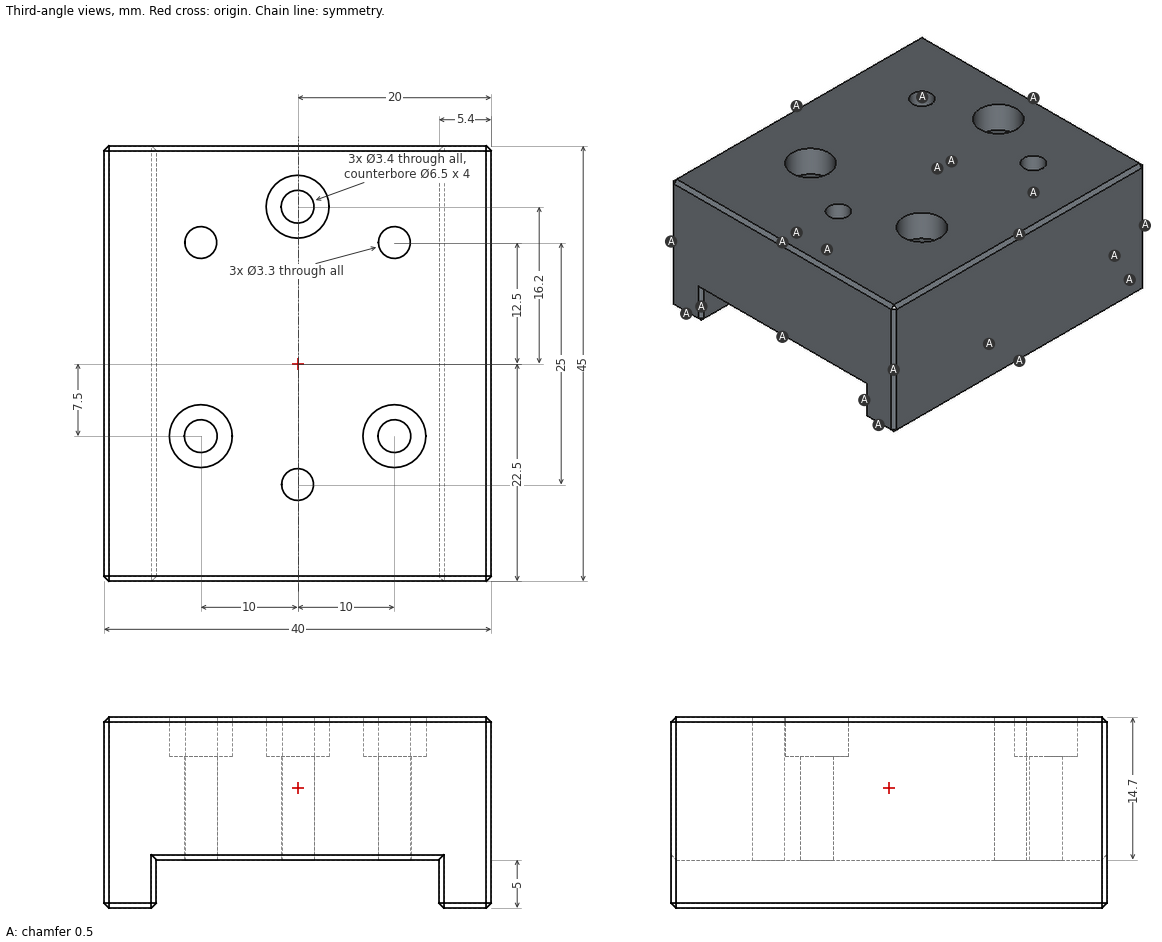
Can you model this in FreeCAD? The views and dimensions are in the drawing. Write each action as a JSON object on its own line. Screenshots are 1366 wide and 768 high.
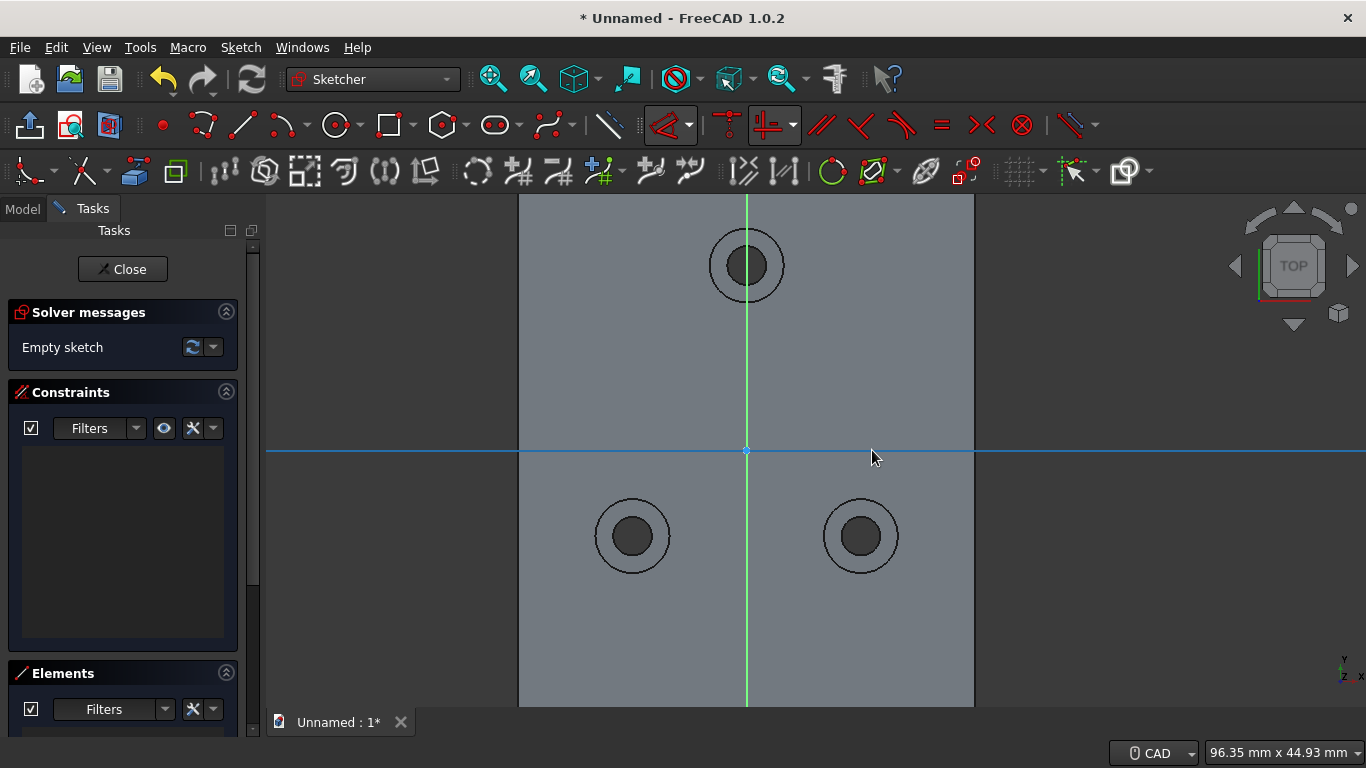
{"action": "left_click", "coordinate": [336, 126]}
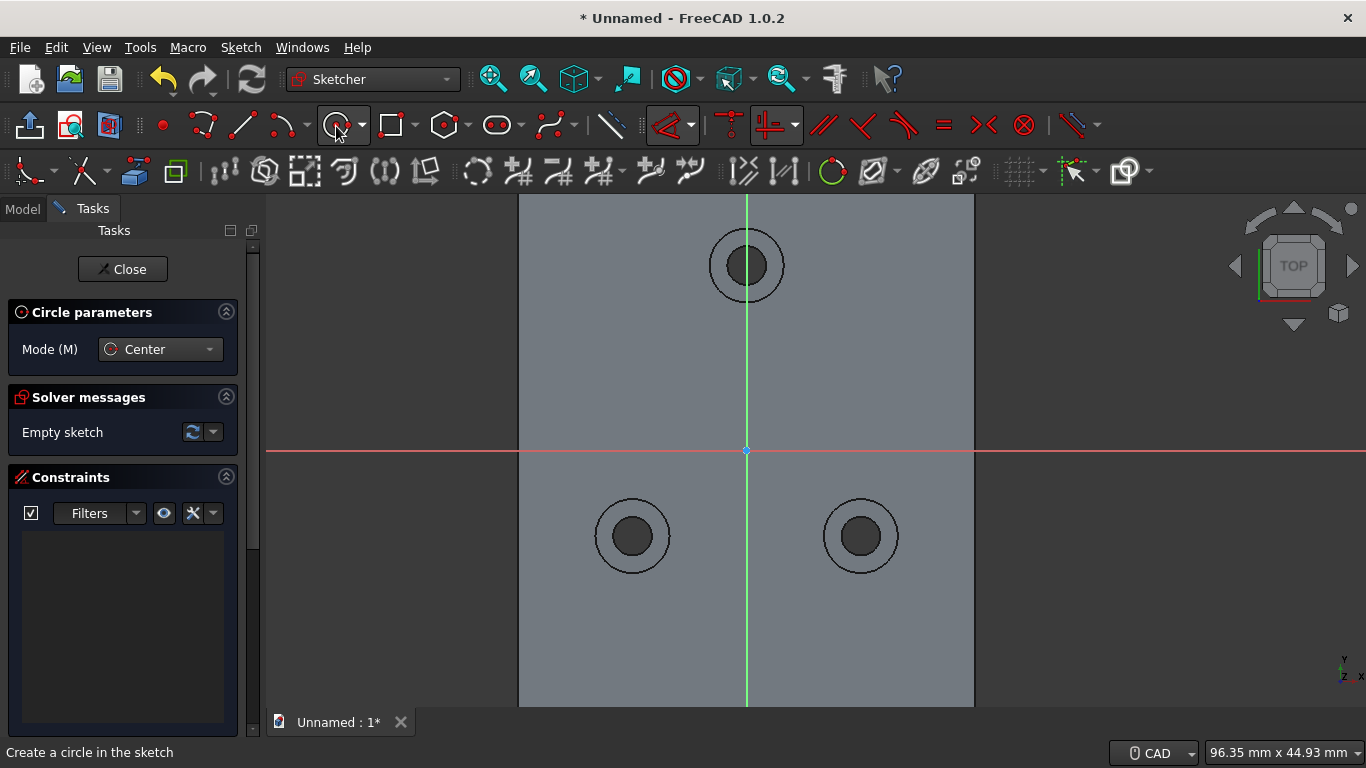
{"action": "left_click", "coordinate": [861, 308]}
{"action": "left_click", "coordinate": [874, 294]}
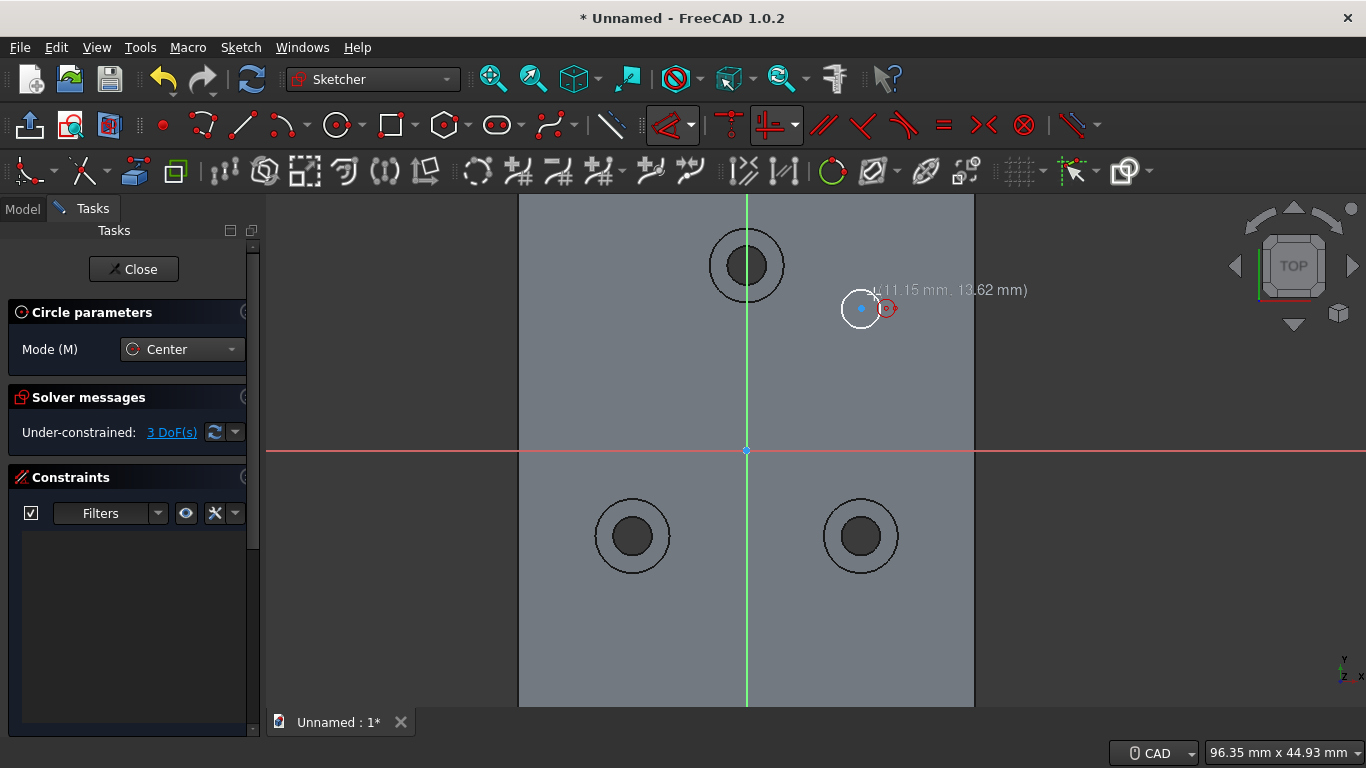
{"action": "left_click", "coordinate": [633, 308]}
{"action": "left_click", "coordinate": [646, 294]}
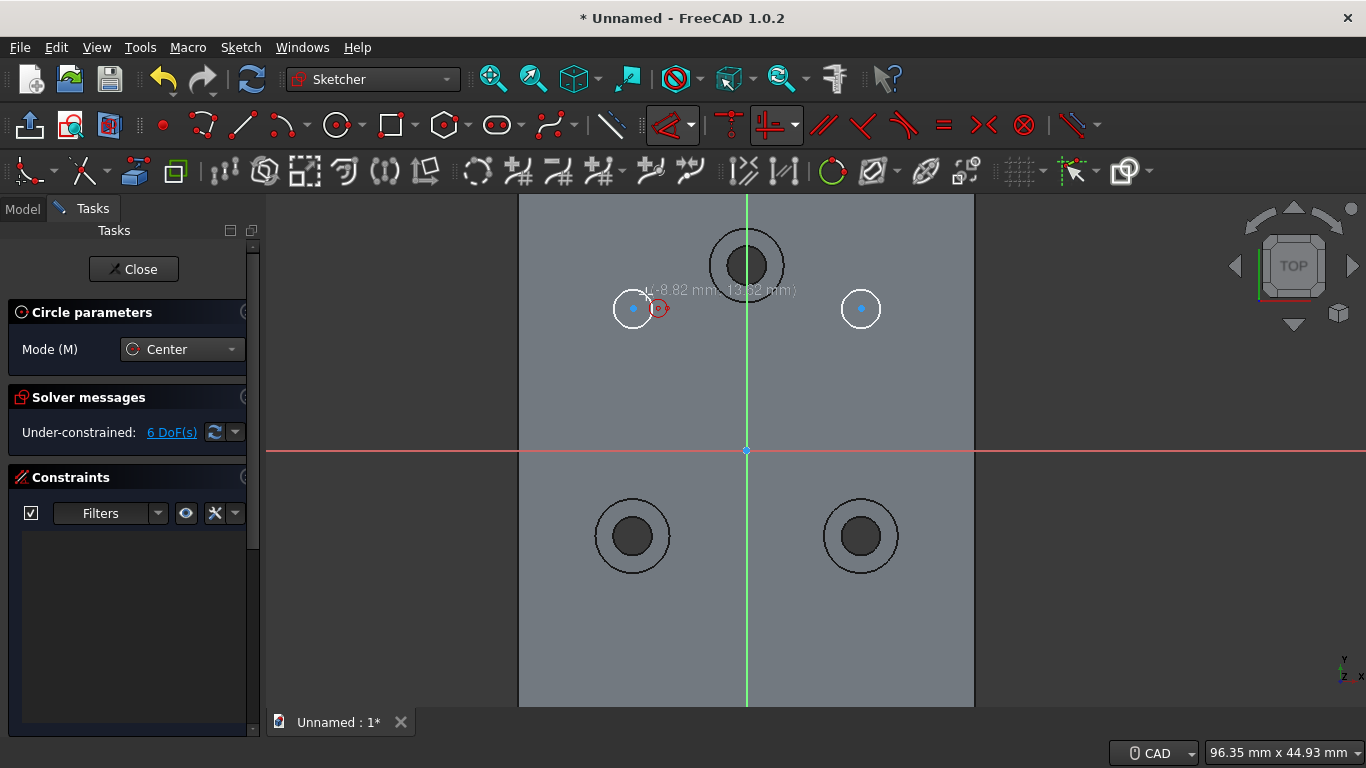
{"action": "left_click", "coordinate": [747, 593]}
{"action": "left_click", "coordinate": [764, 587]}
{"action": "key", "text": "Escape"}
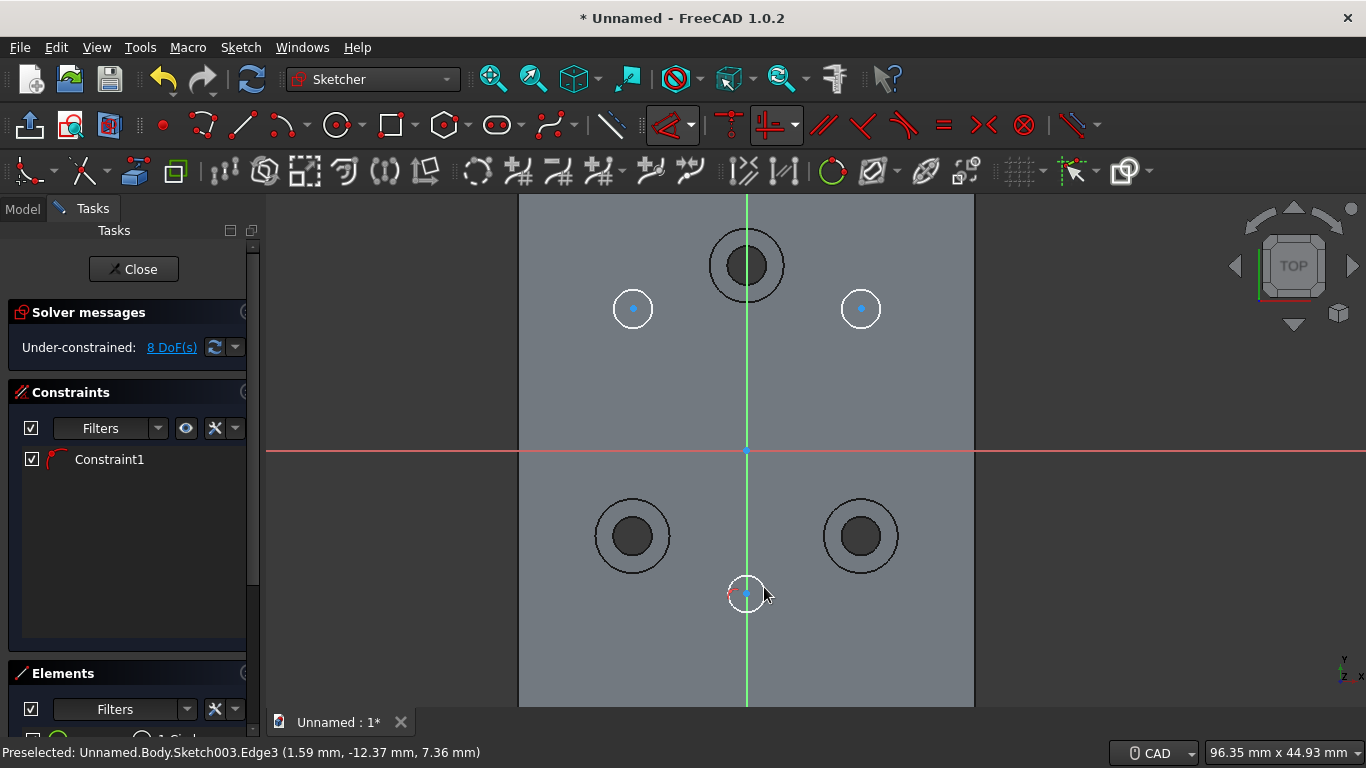
{"action": "left_click", "coordinate": [874, 295]}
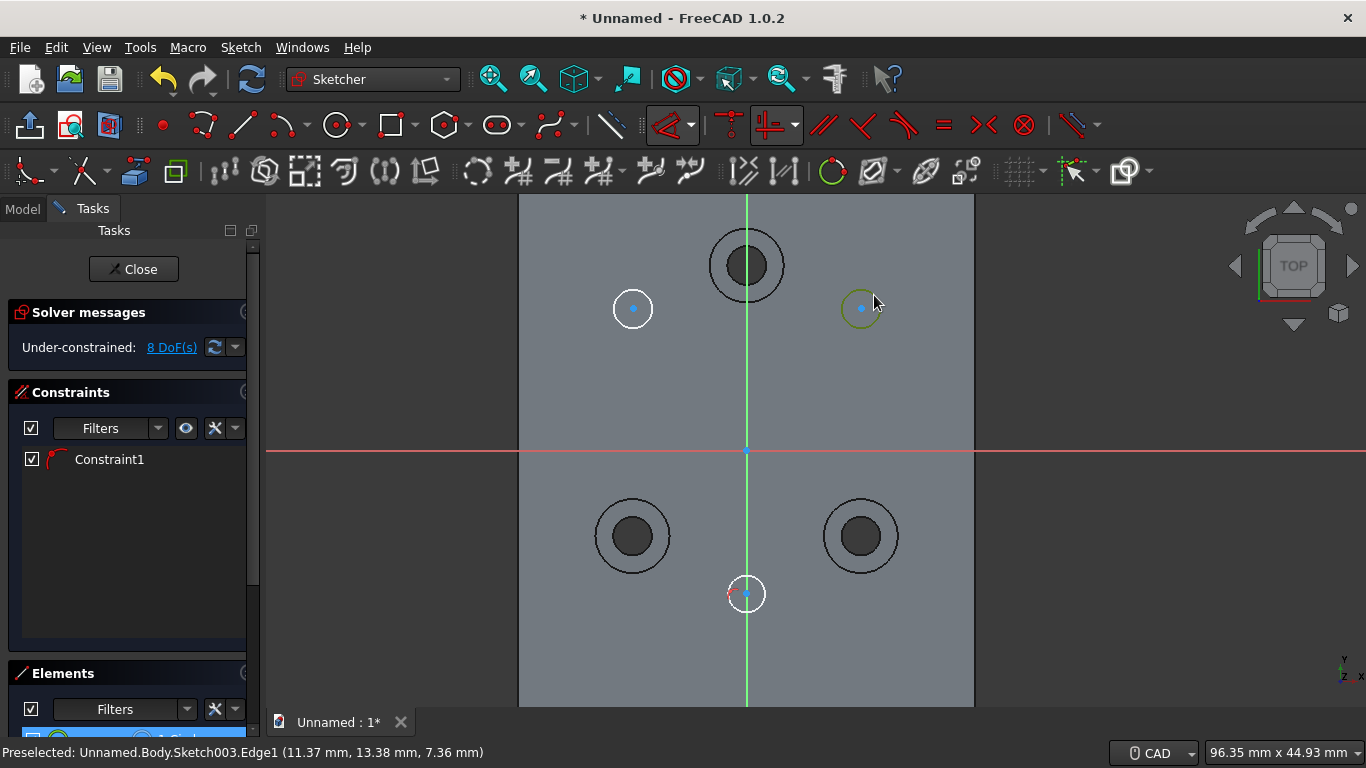
{"action": "left_click", "coordinate": [646, 295]}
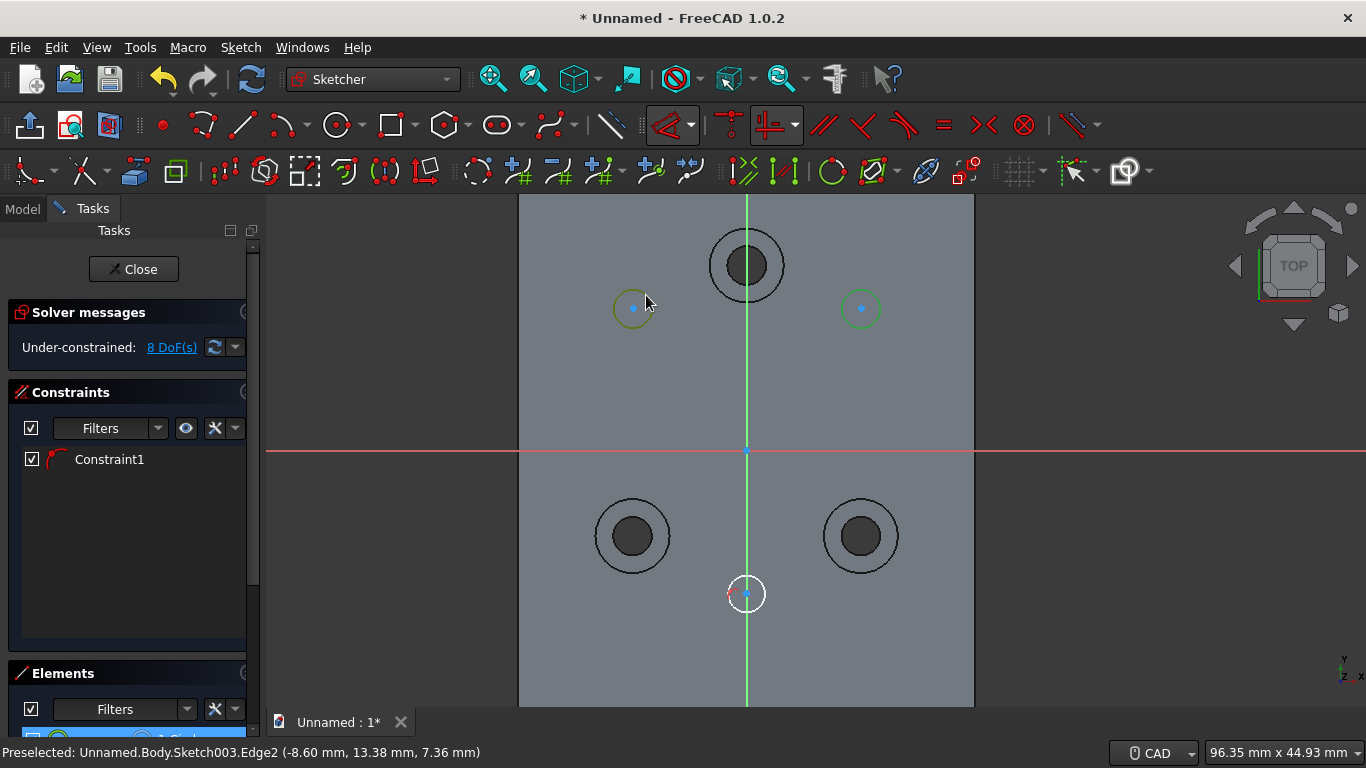
{"action": "left_click", "coordinate": [760, 581]}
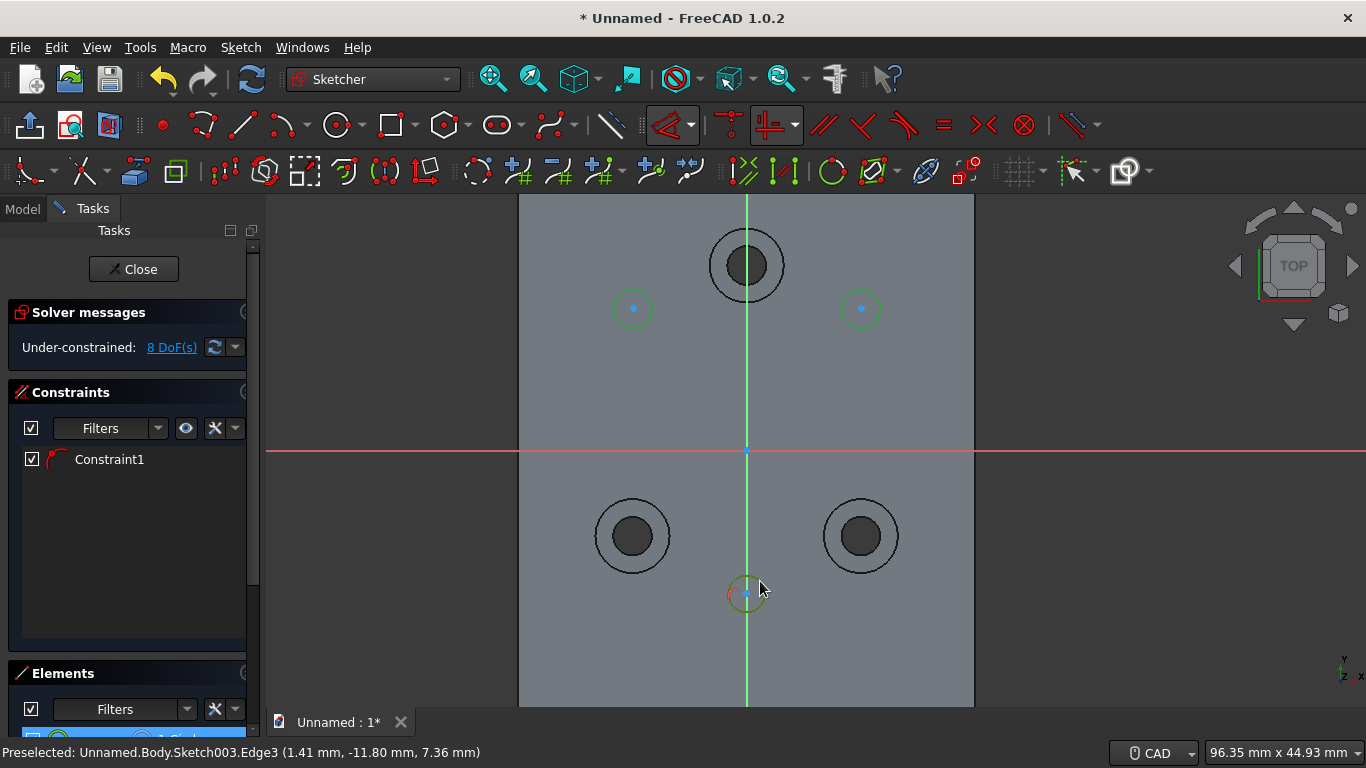
{"action": "key", "text": "e"}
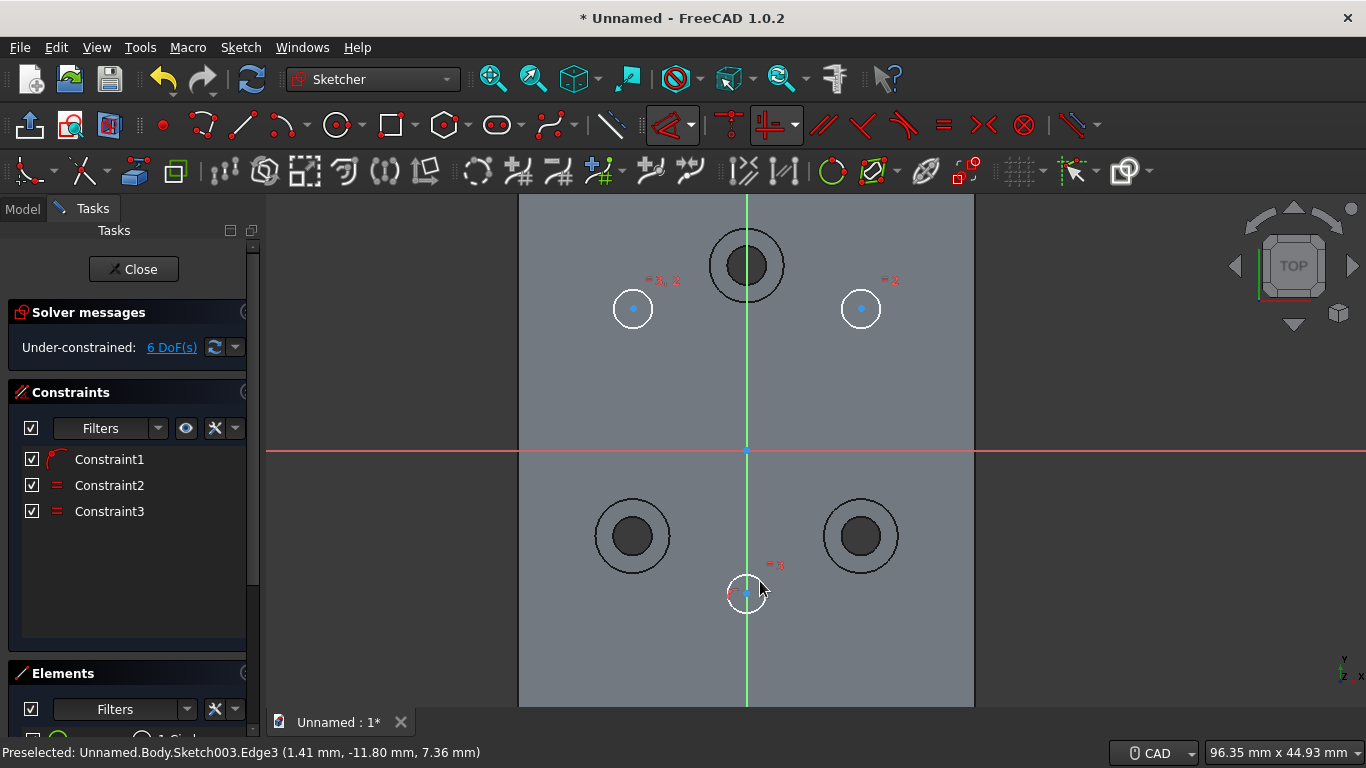
{"action": "left_click", "coordinate": [861, 309]}